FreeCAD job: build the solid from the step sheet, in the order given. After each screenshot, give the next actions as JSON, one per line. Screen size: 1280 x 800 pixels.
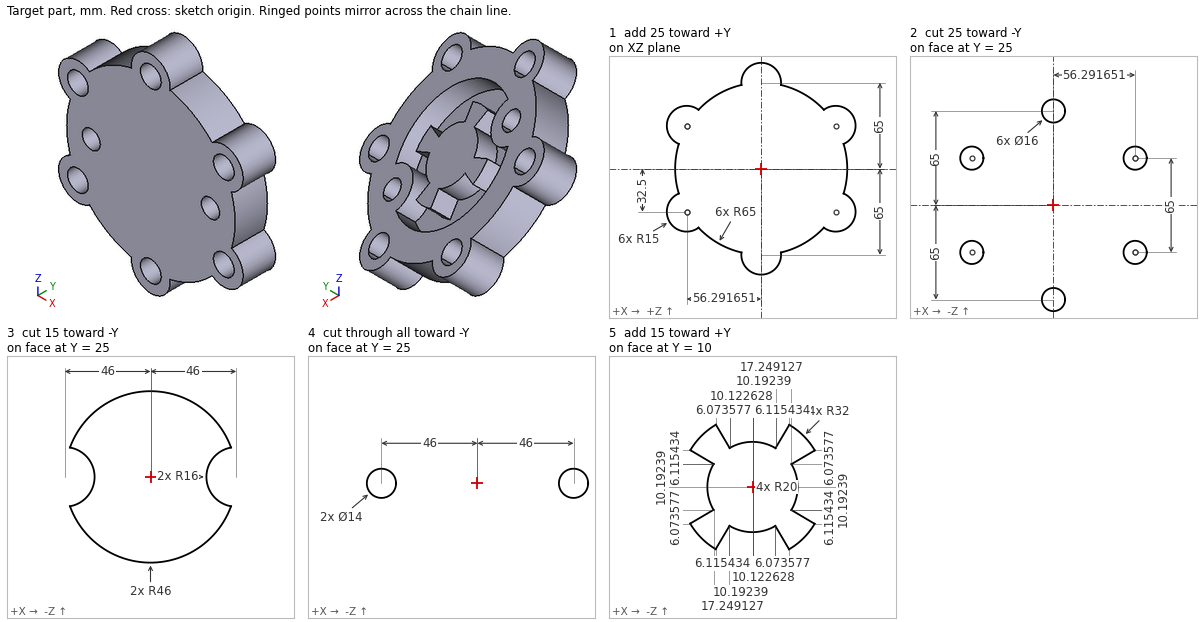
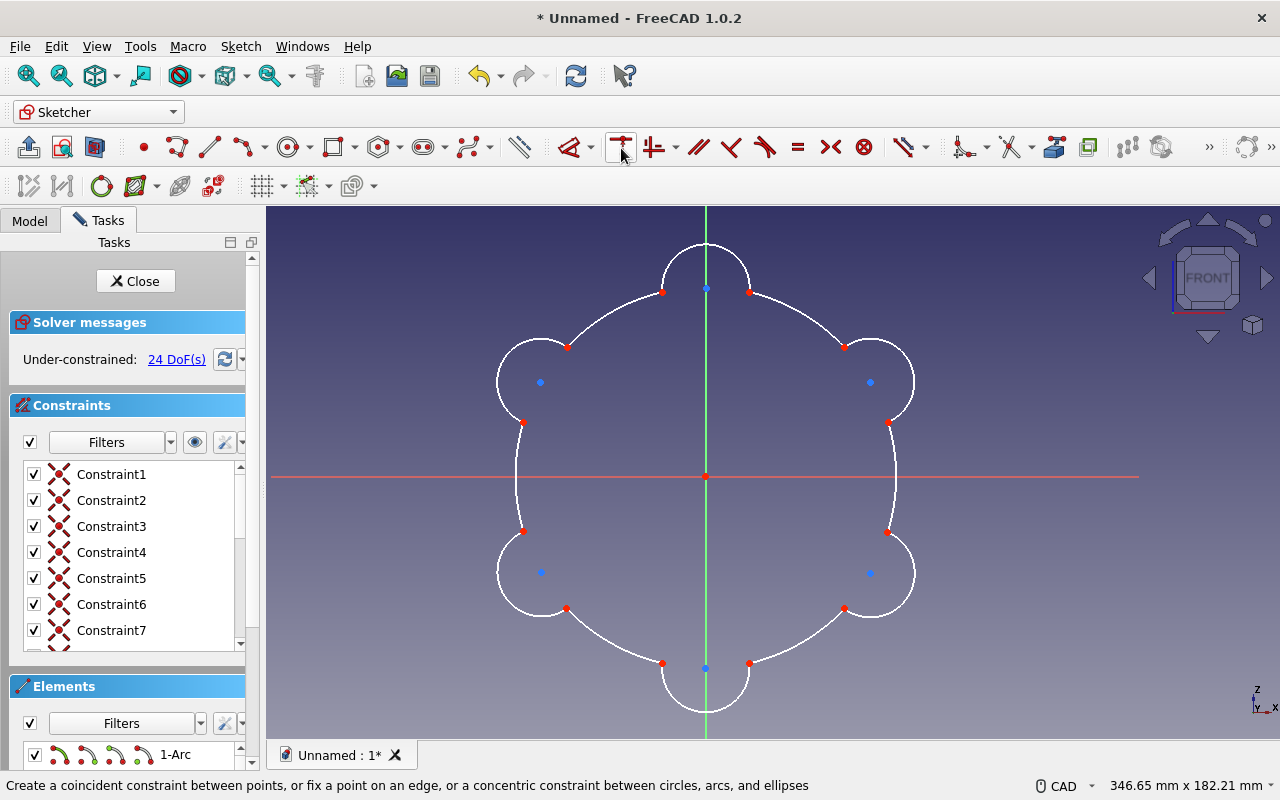
{"action": "left_click", "coordinate": [592, 631]}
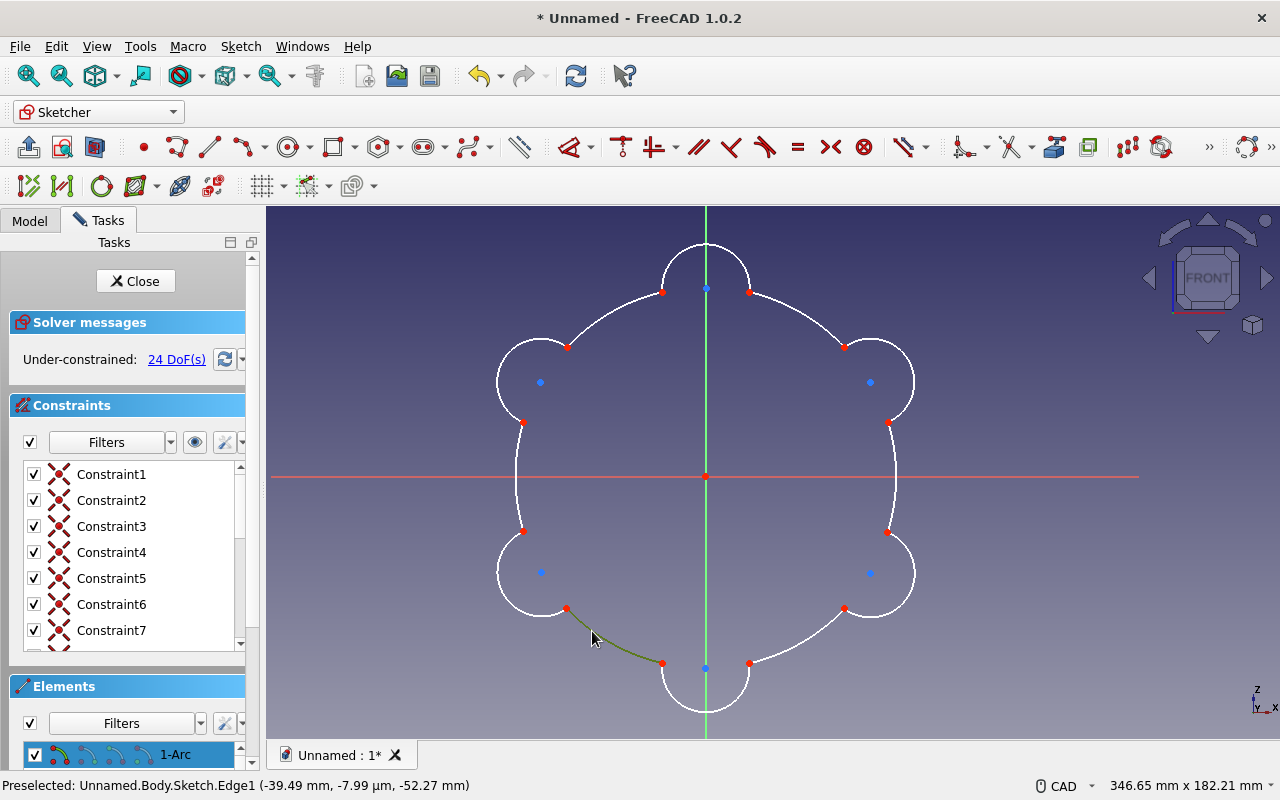
{"action": "left_click", "coordinate": [517, 455]}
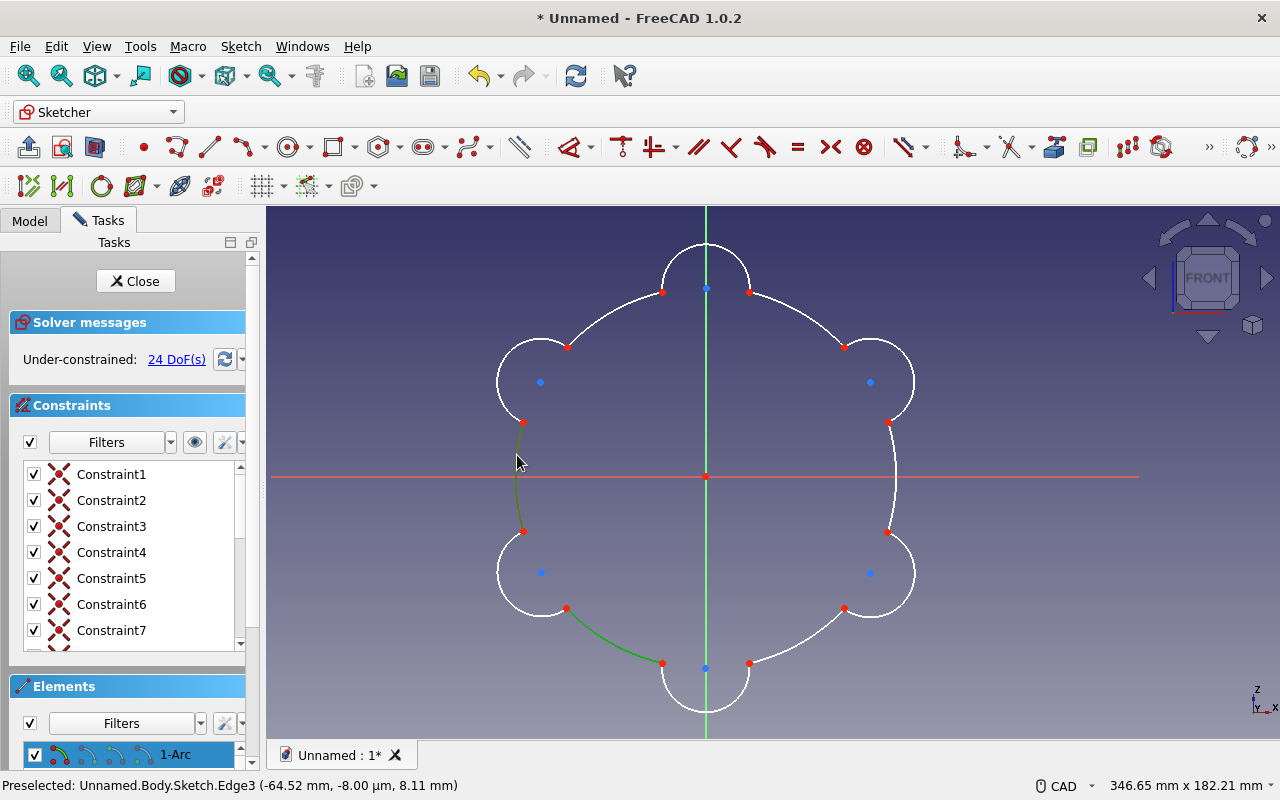
{"action": "left_click", "coordinate": [631, 303]}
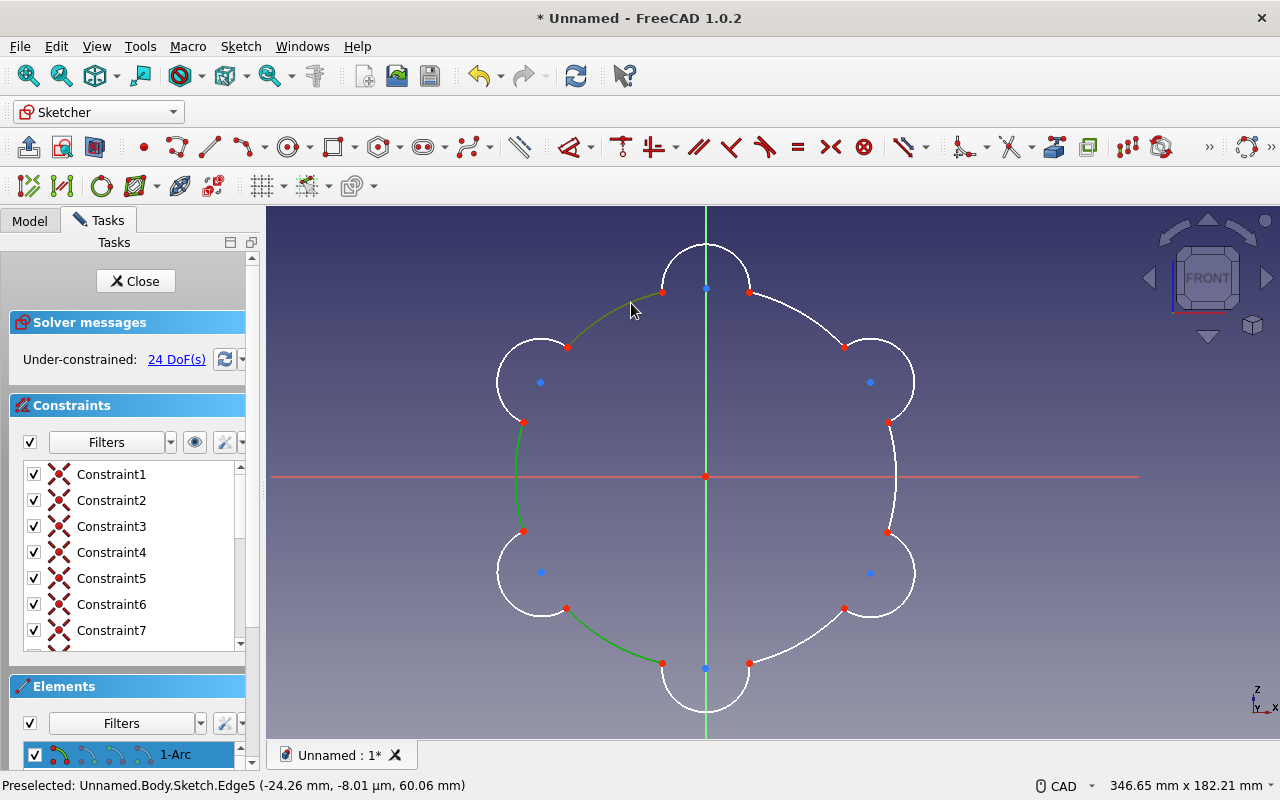
{"action": "left_click", "coordinate": [820, 325]}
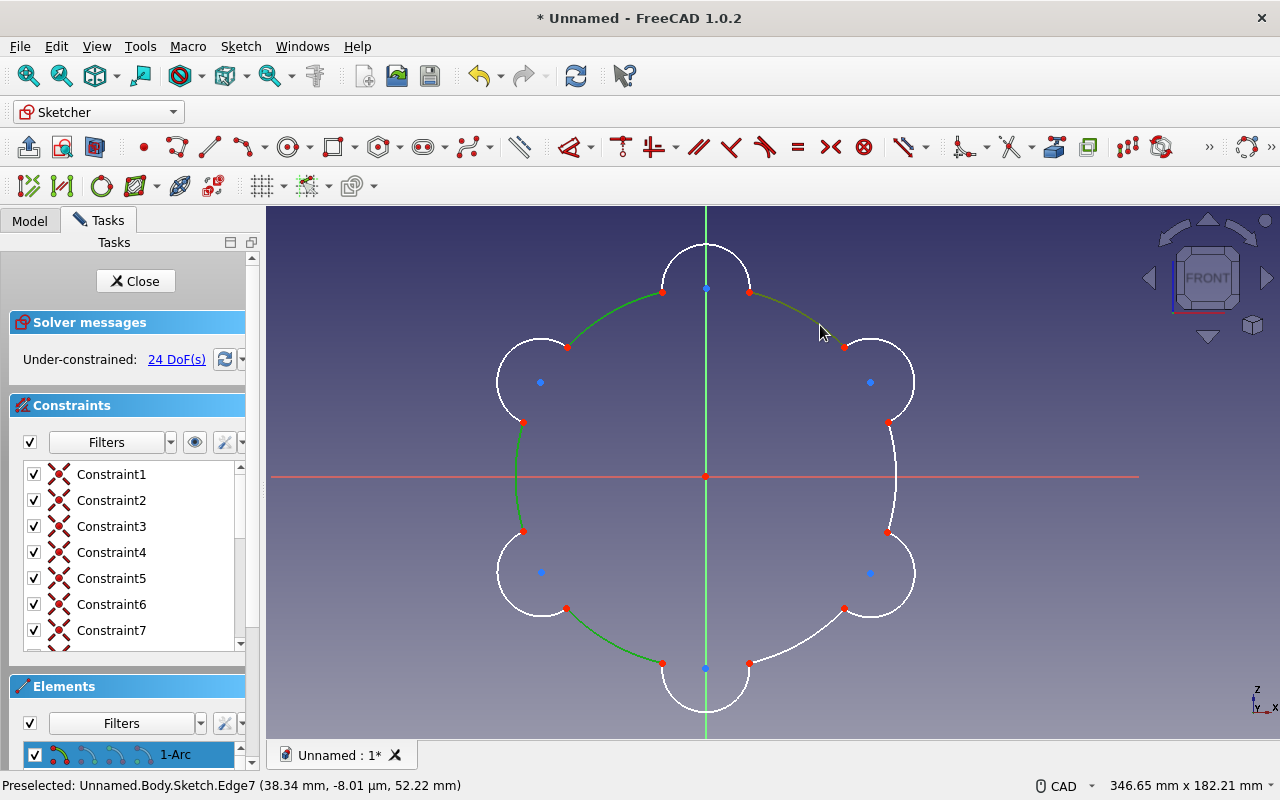
{"action": "left_click", "coordinate": [895, 500]}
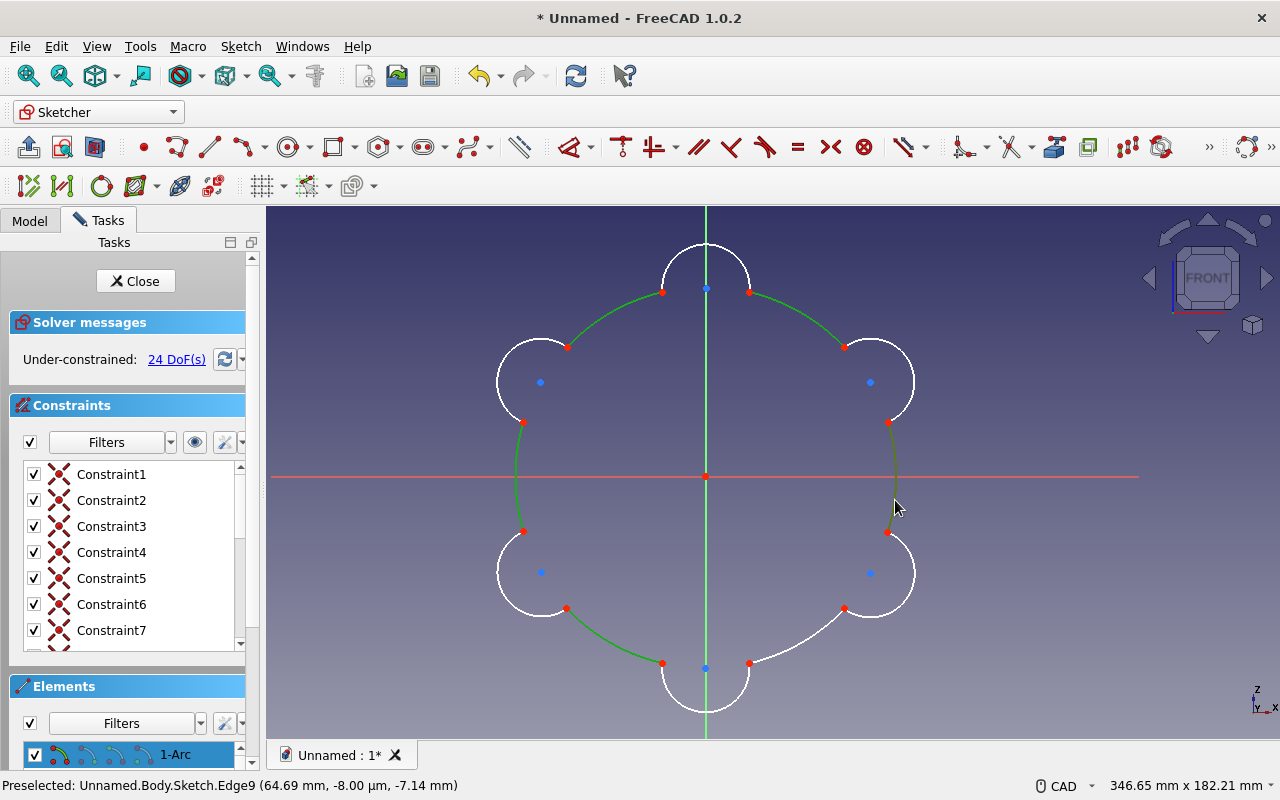
{"action": "left_click", "coordinate": [781, 653]}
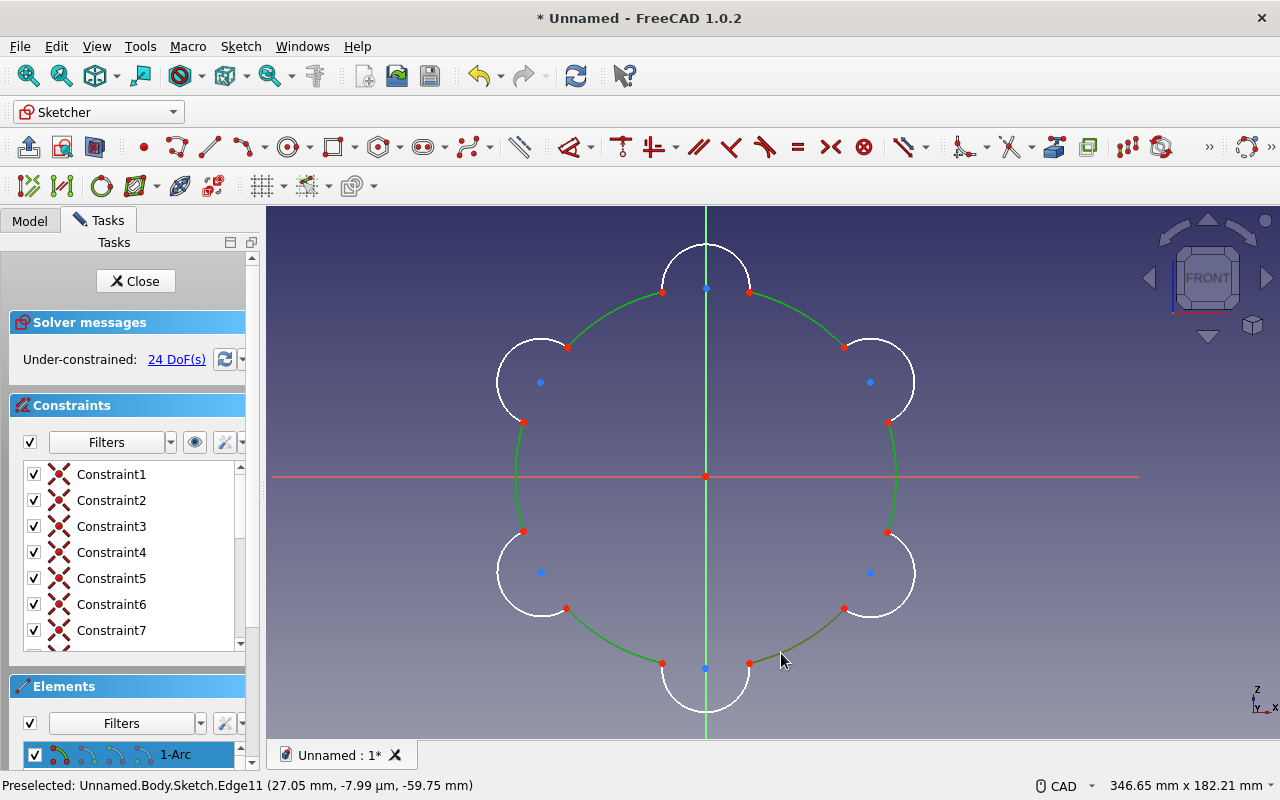
{"action": "left_click", "coordinate": [798, 148]}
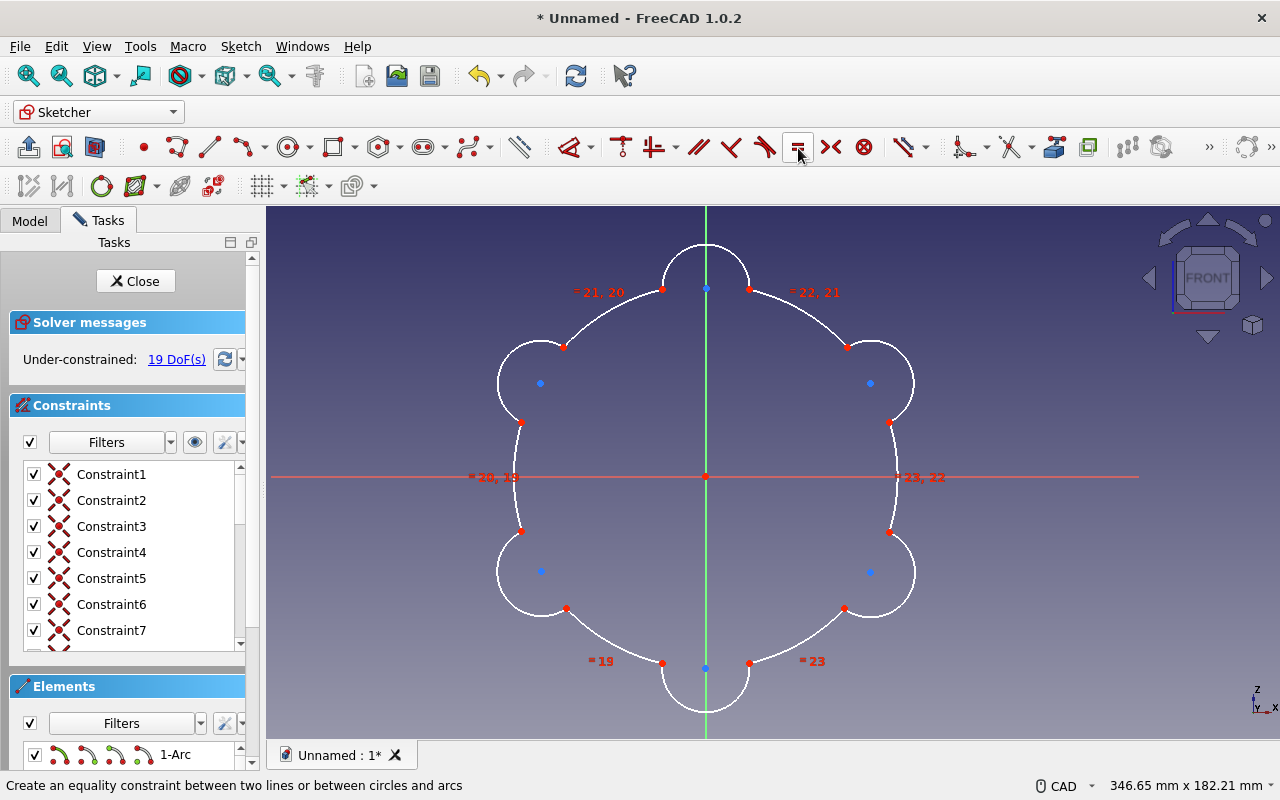
{"action": "left_click", "coordinate": [498, 566]}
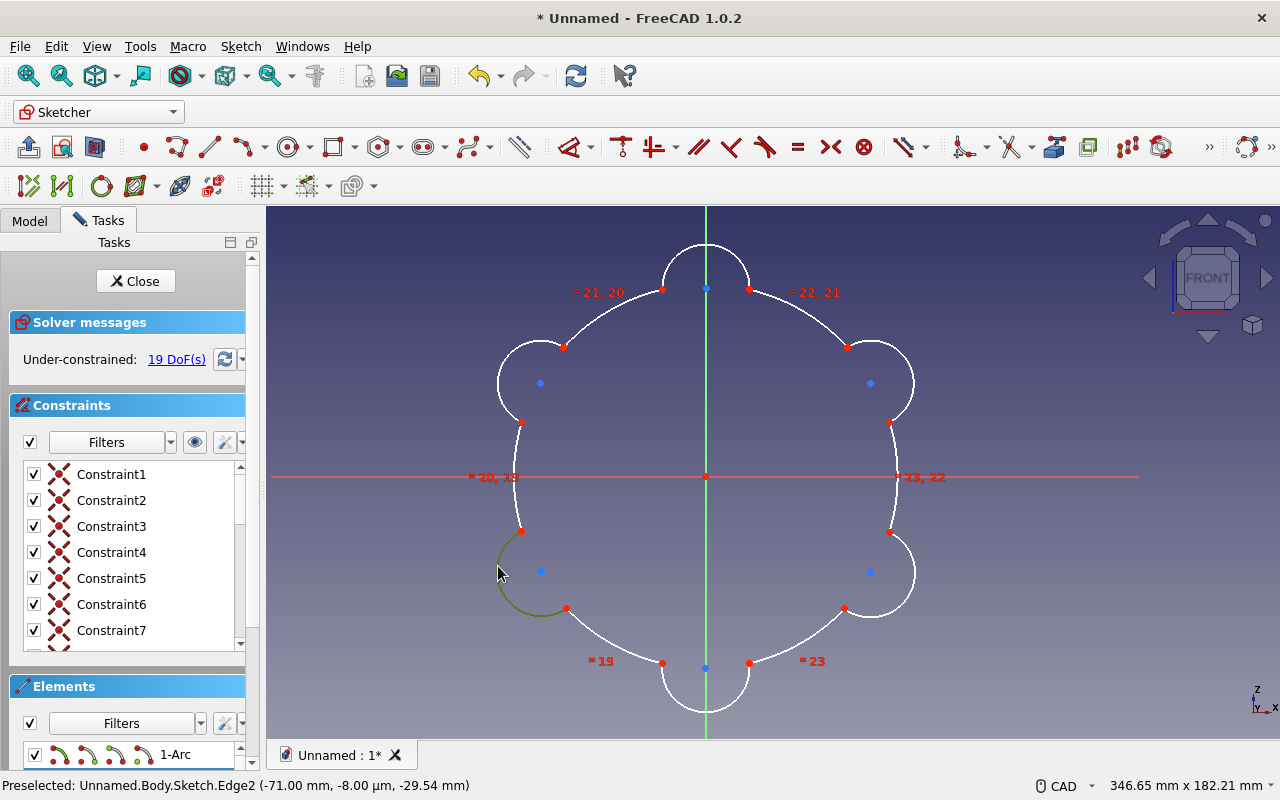
{"action": "left_click", "coordinate": [524, 344]}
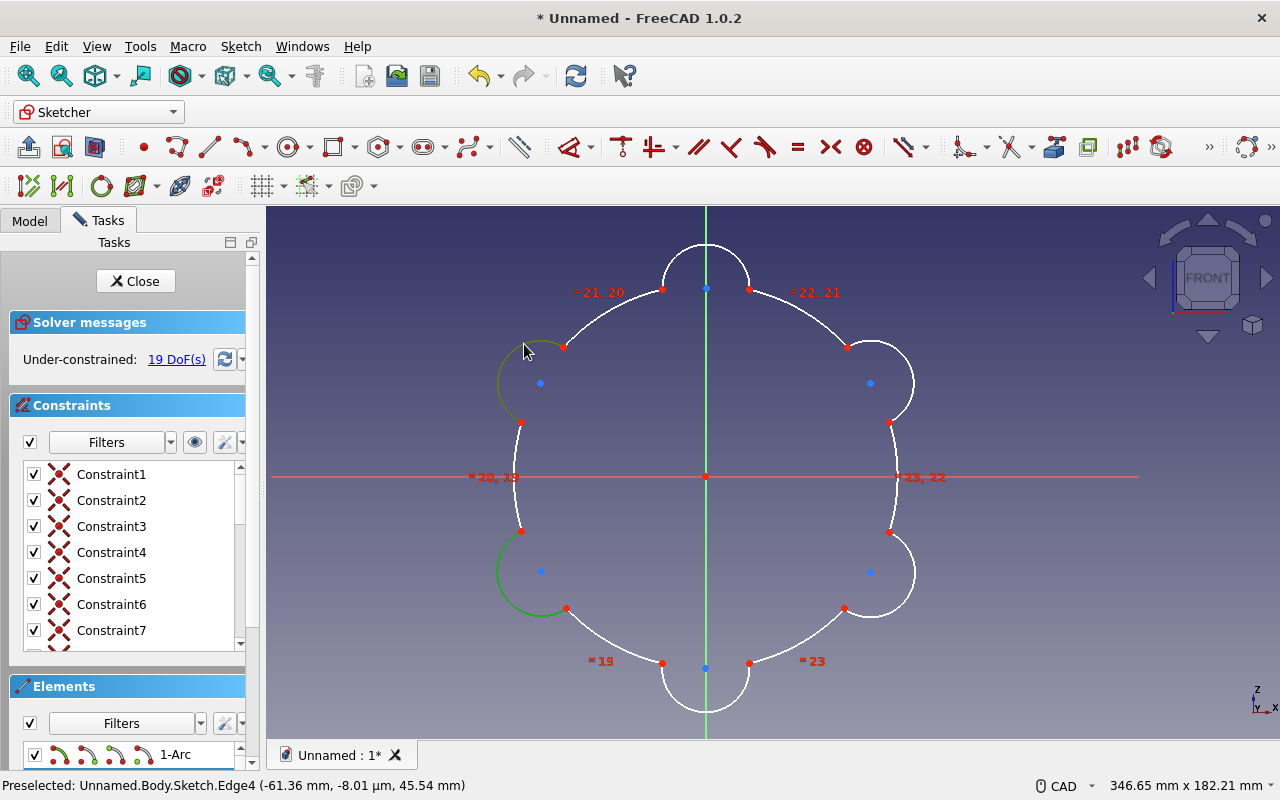
{"action": "left_click", "coordinate": [732, 253]}